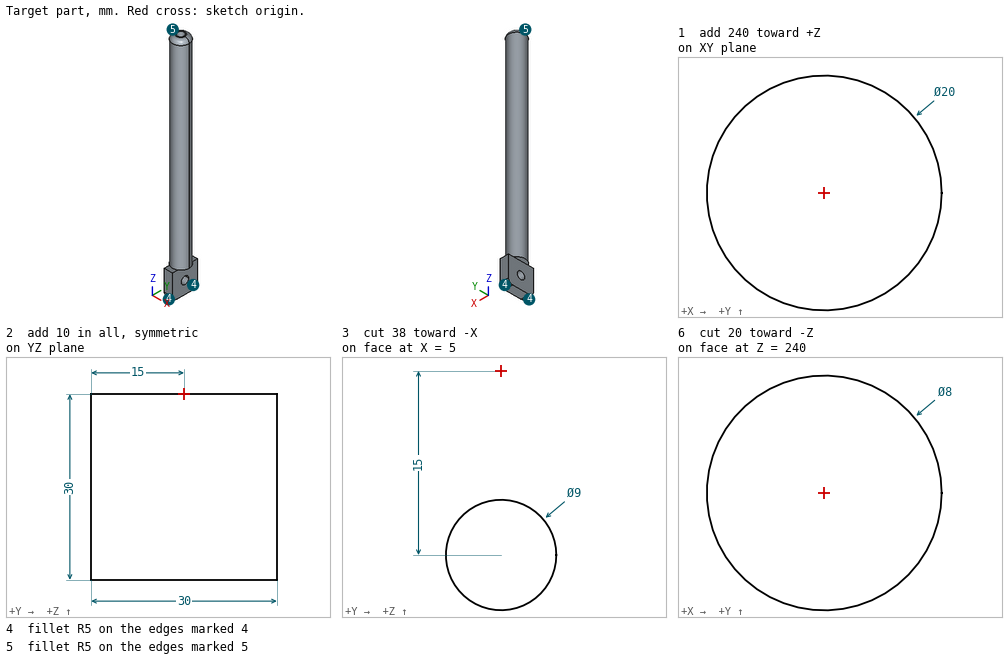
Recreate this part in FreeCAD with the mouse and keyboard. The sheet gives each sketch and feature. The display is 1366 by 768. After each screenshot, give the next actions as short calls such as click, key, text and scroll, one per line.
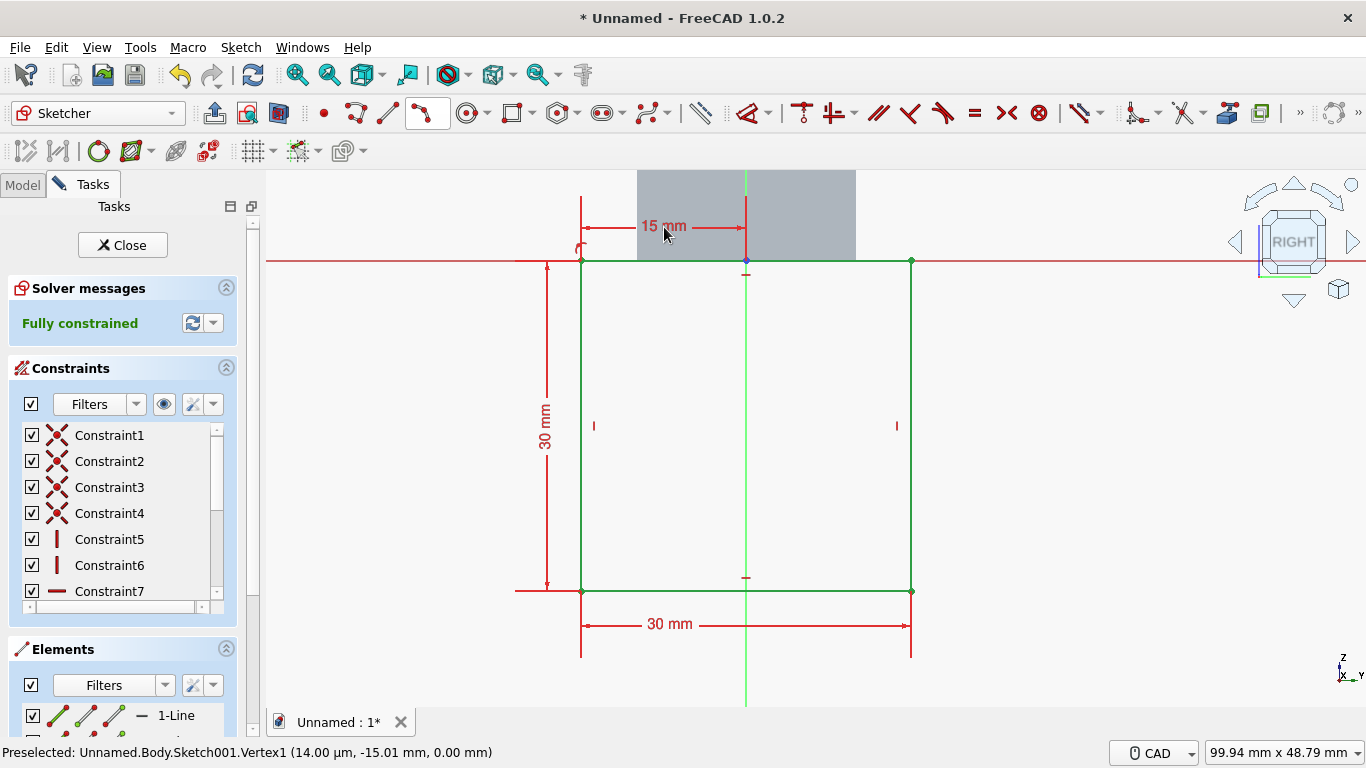
click(123, 245)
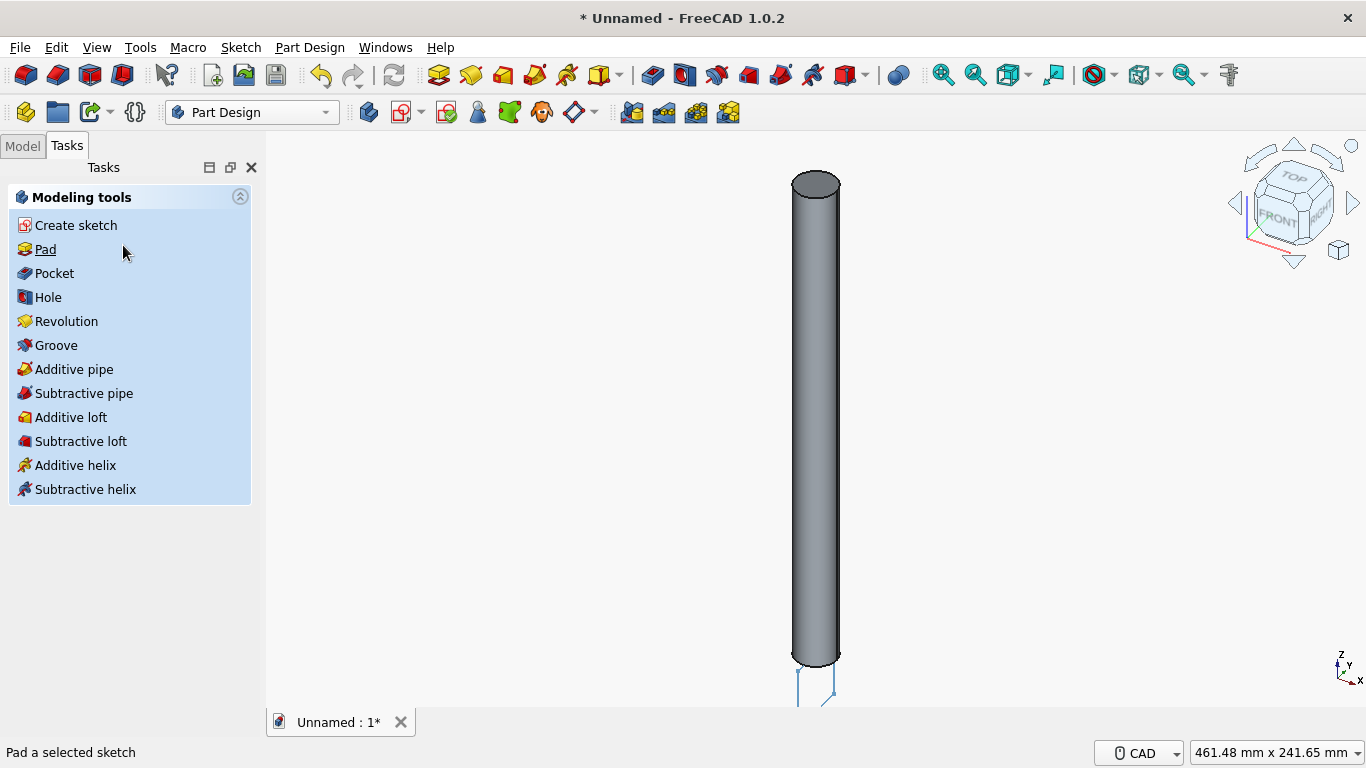
click(440, 76)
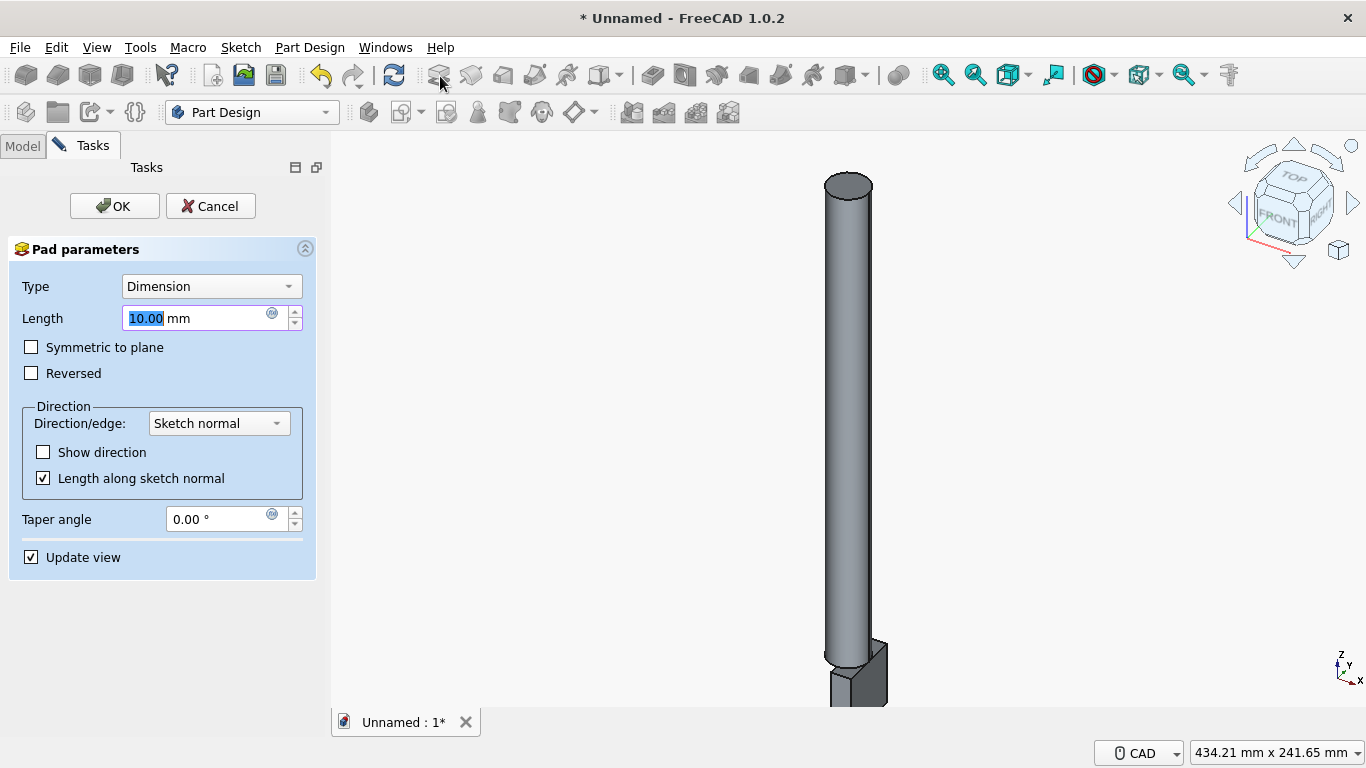
text(10)
key(Tab)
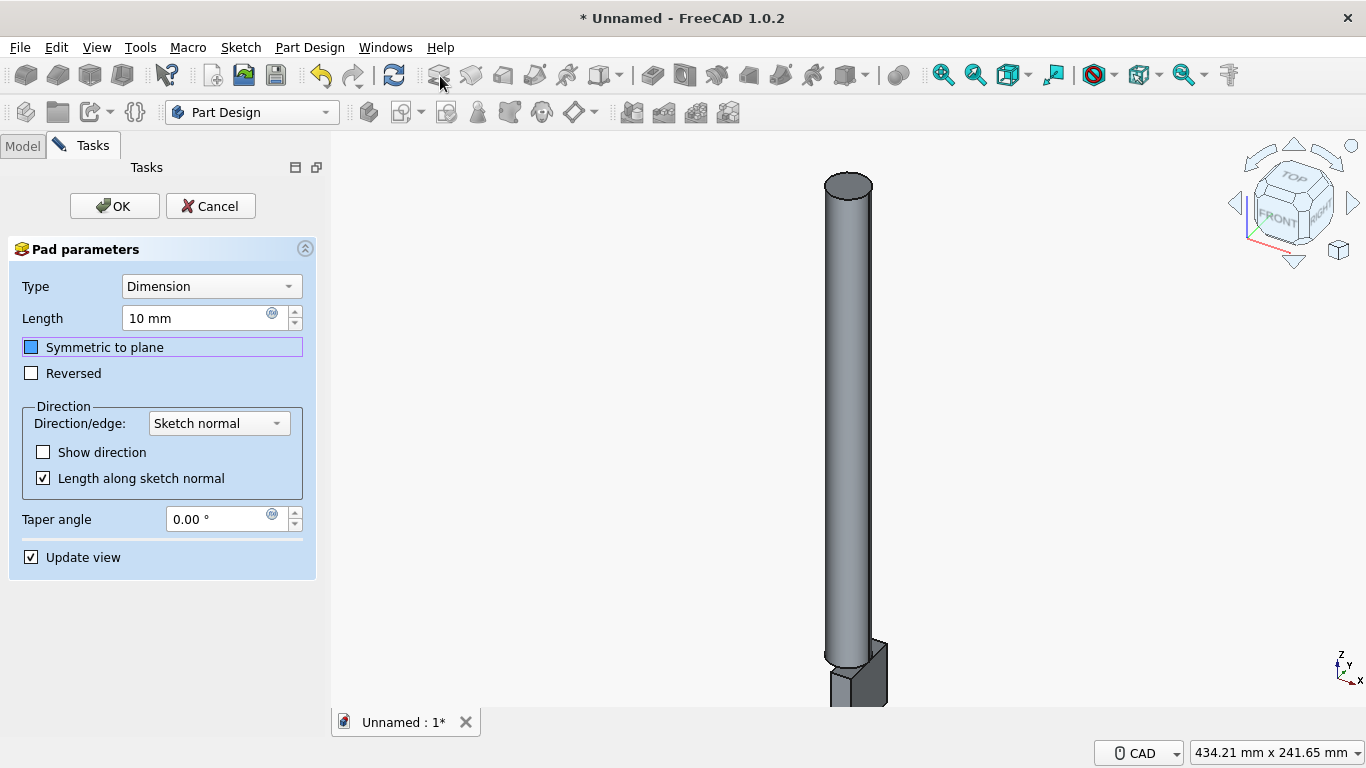
click(30, 347)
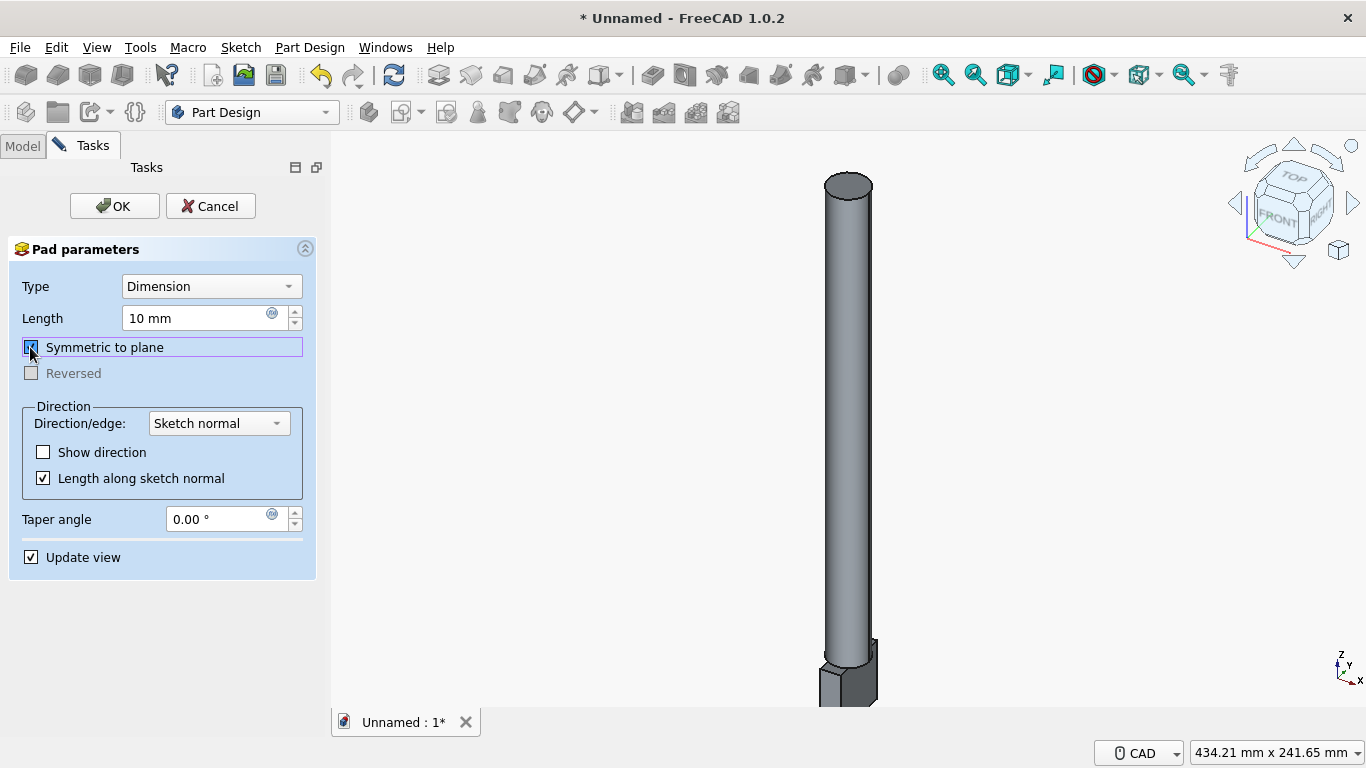
click(115, 206)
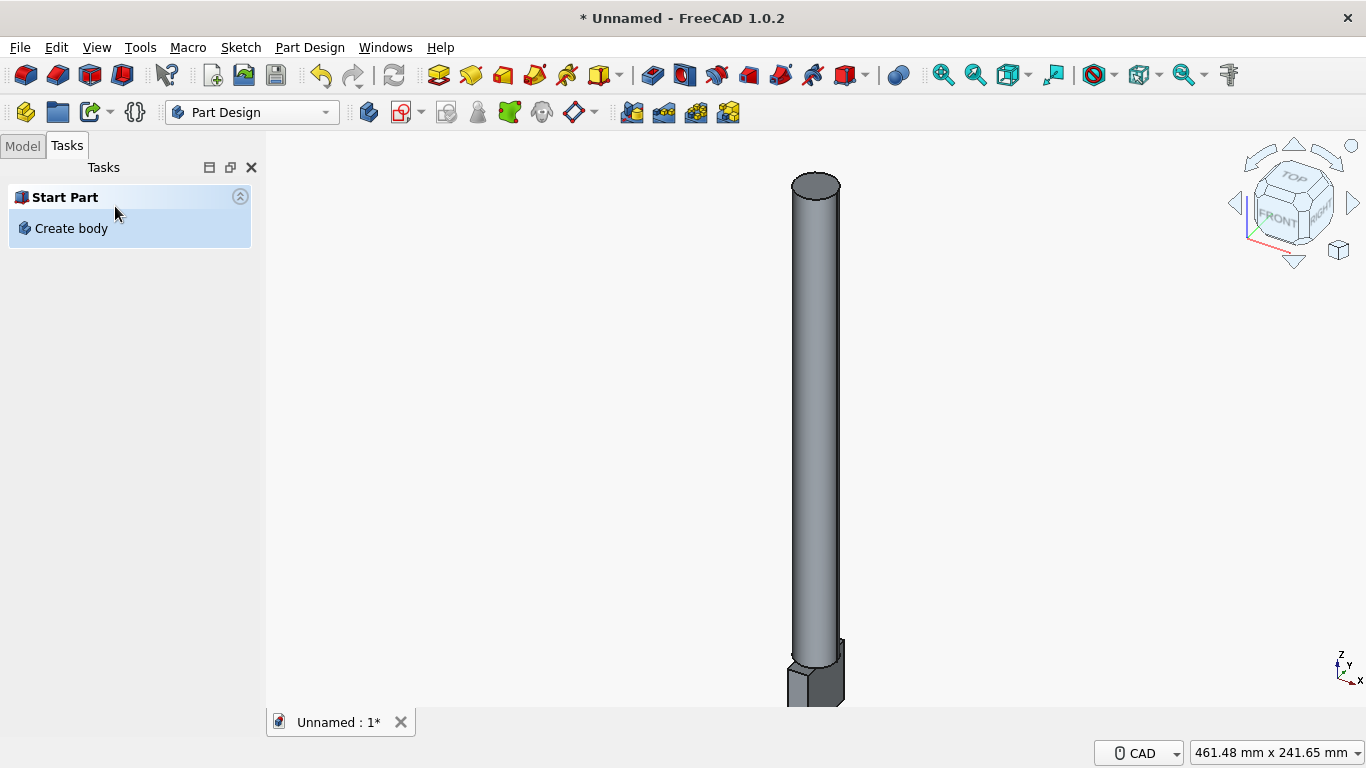
click(944, 76)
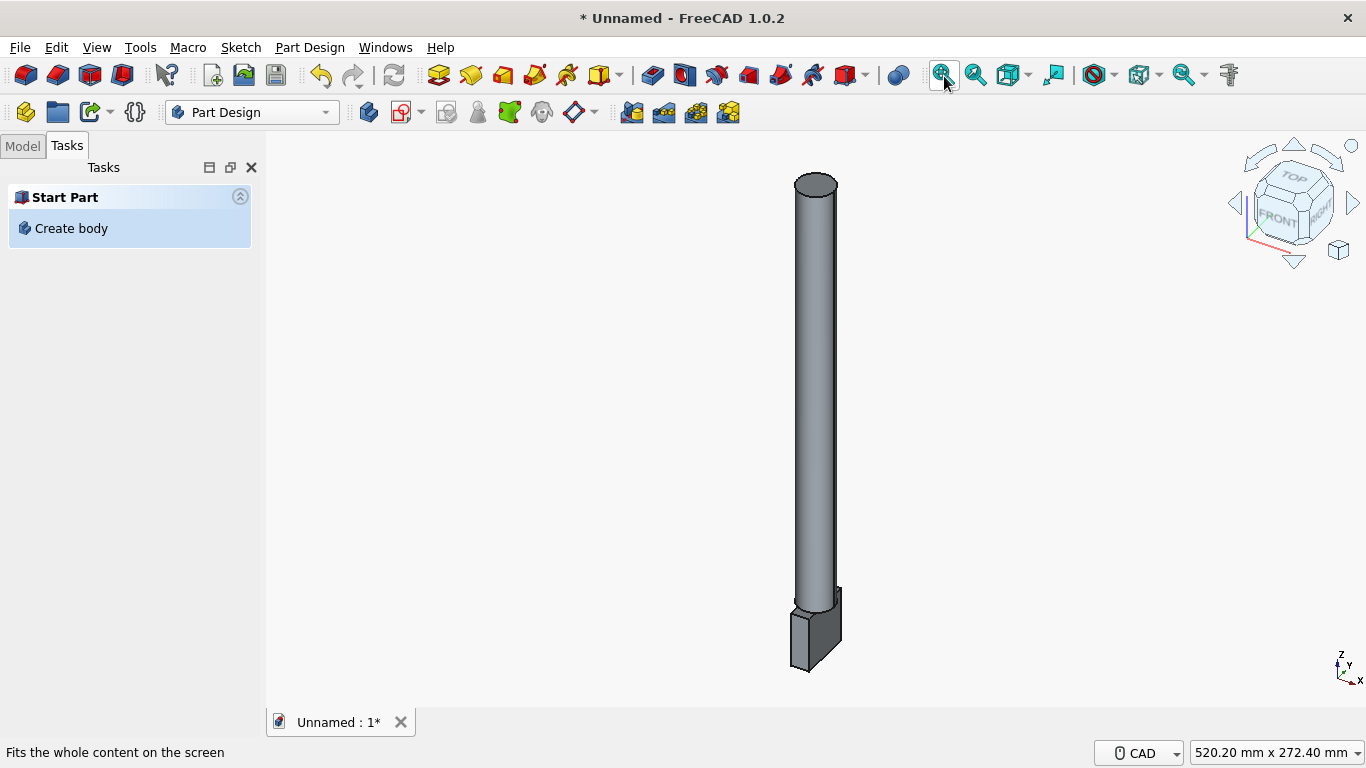
click(825, 629)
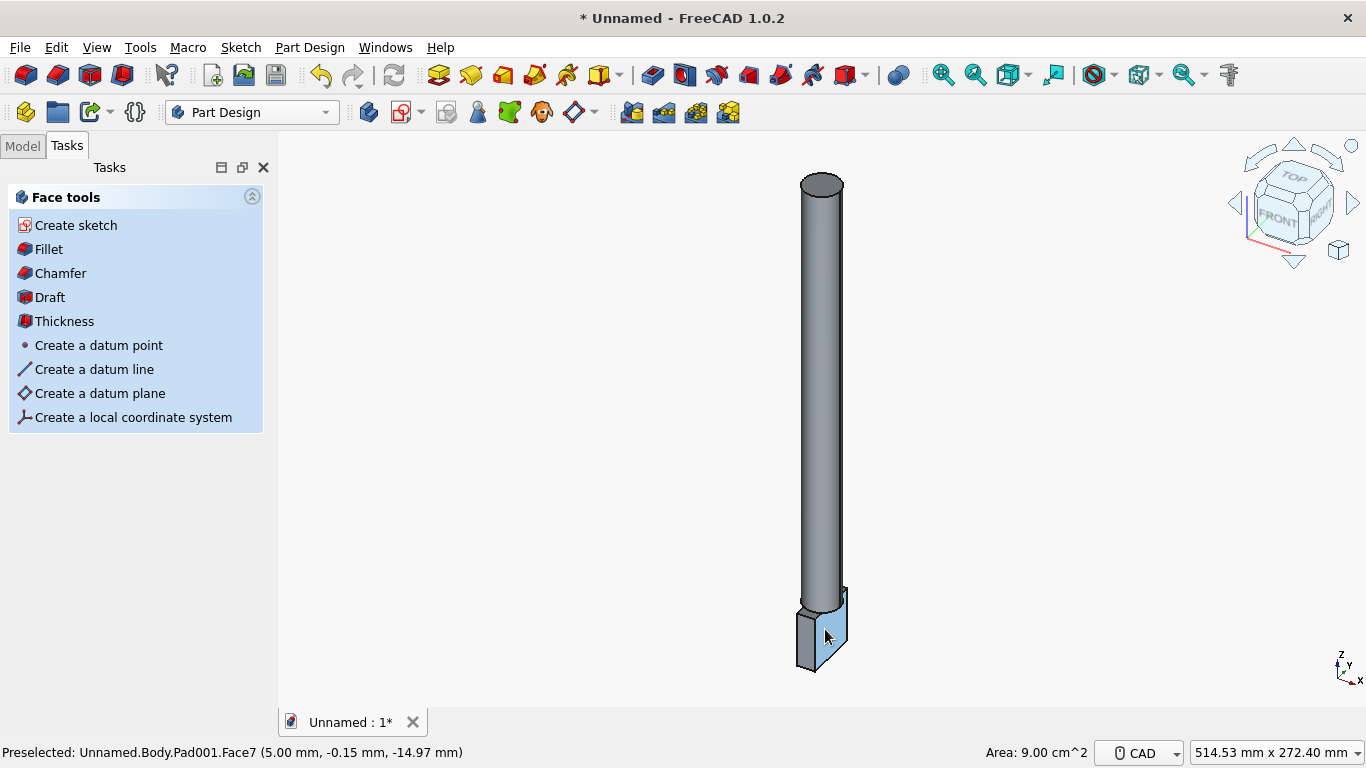
click(402, 112)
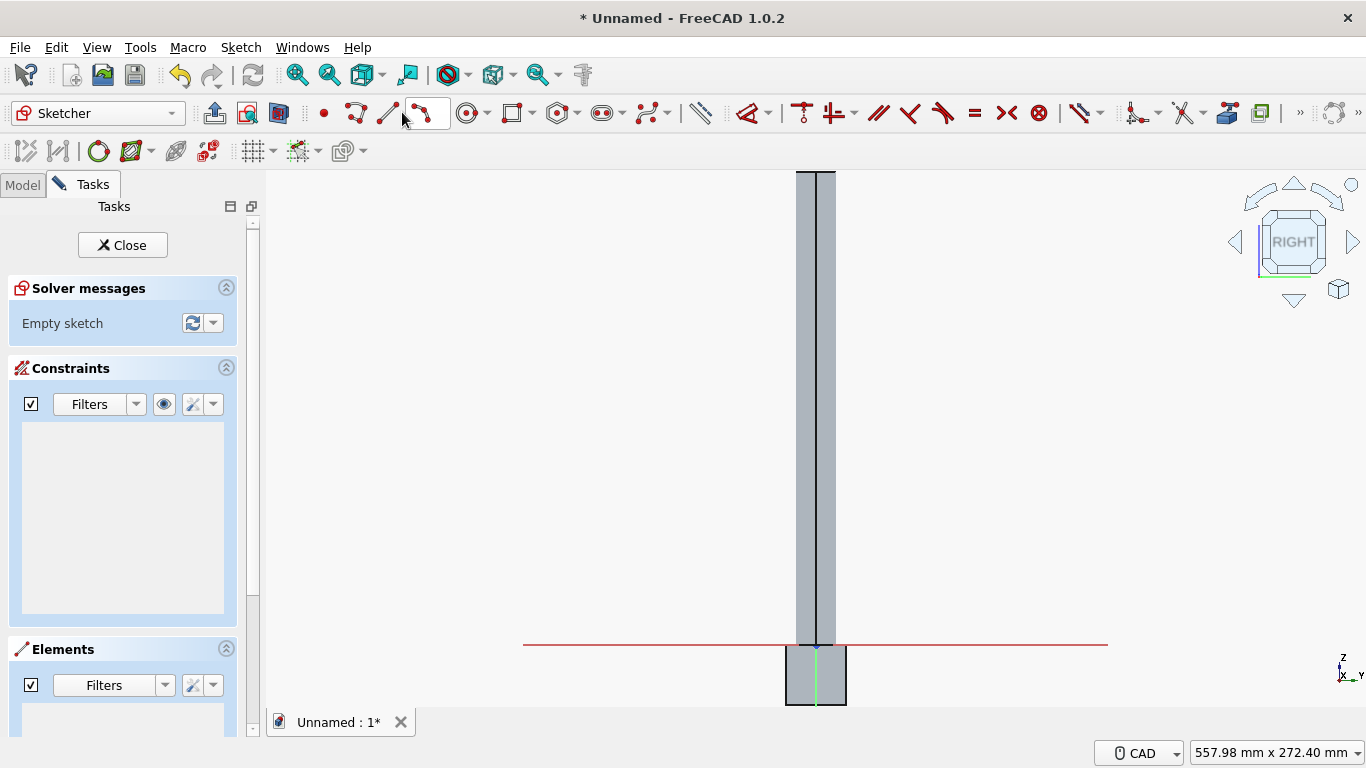
key(q)
key(s)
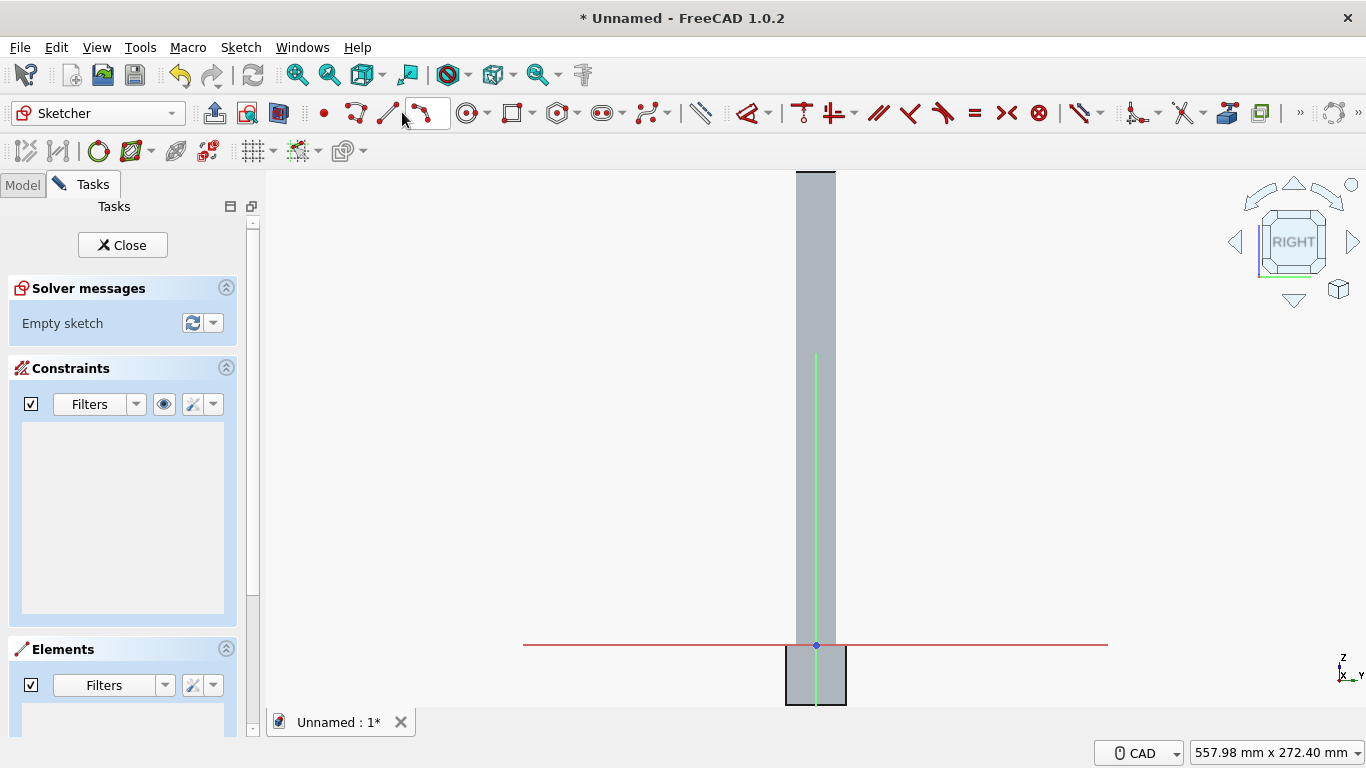
scroll(748, 438, down, 5)